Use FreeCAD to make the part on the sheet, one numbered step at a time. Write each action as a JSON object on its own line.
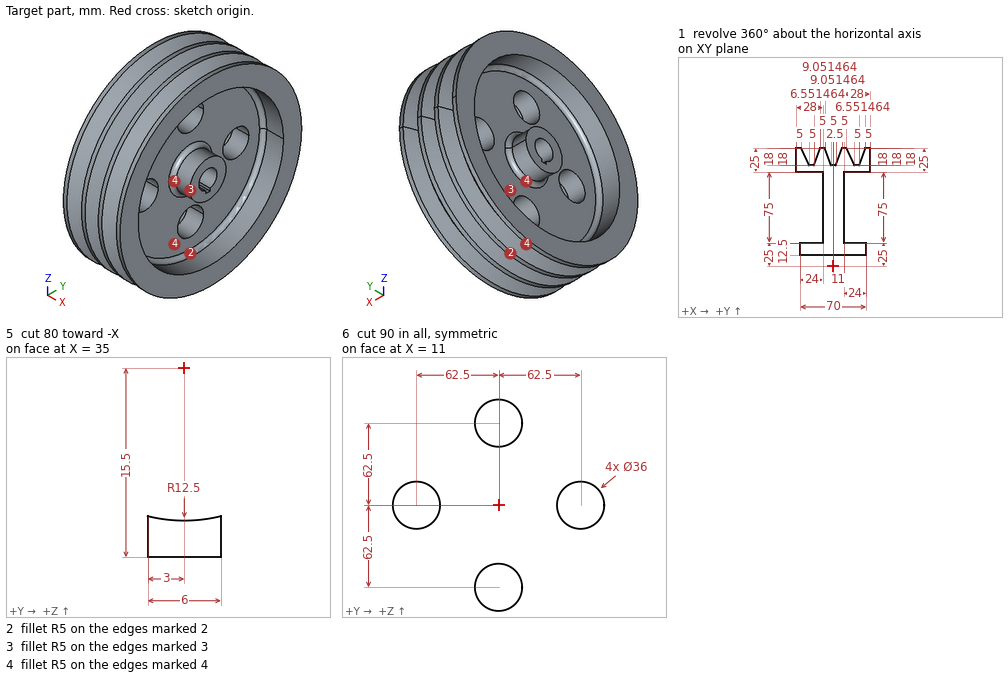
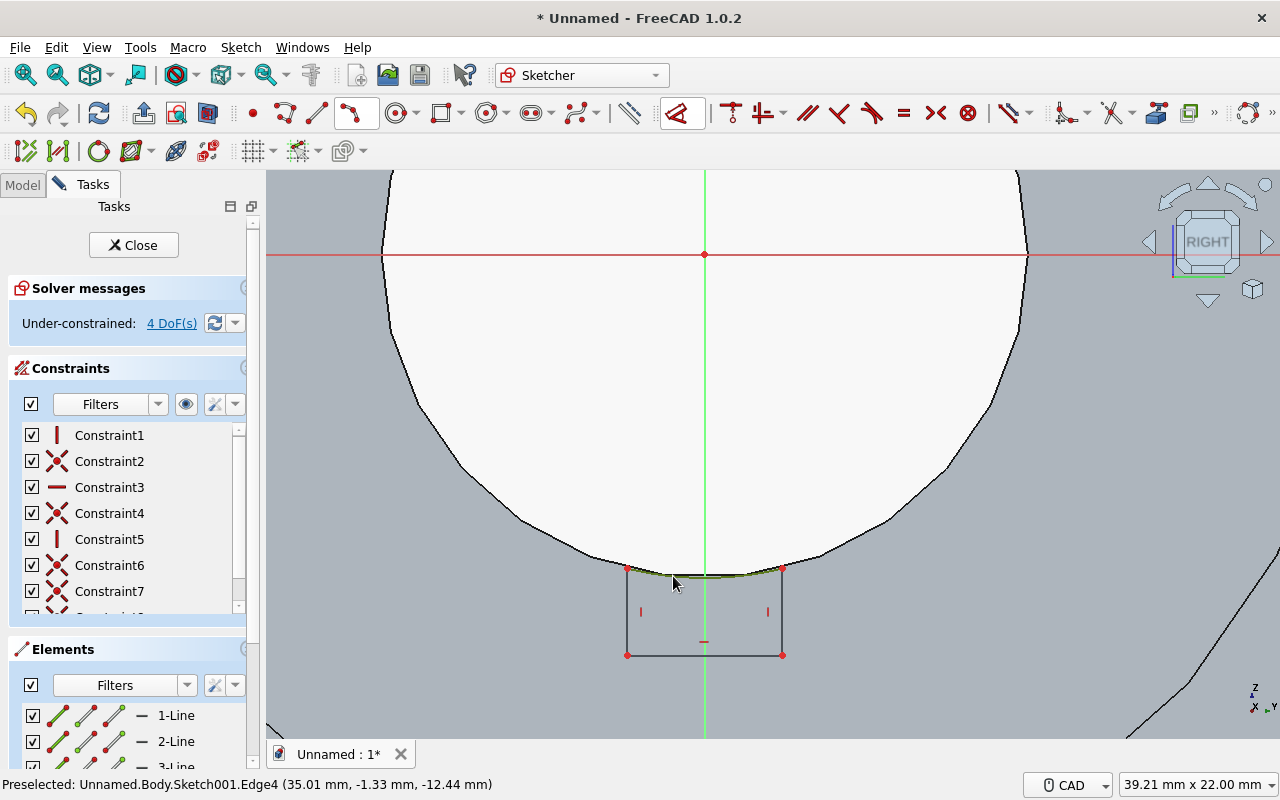
{"action": "left_click", "coordinate": [700, 114]}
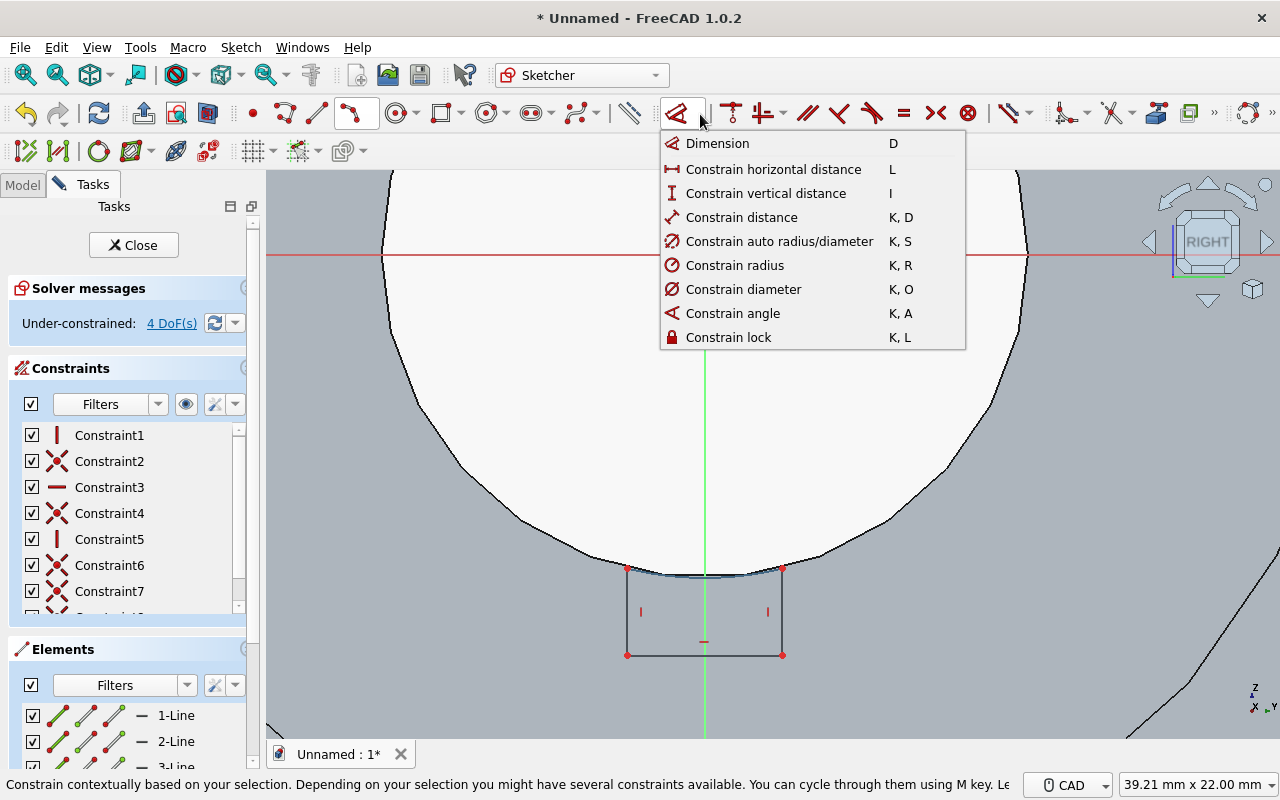
{"action": "left_click", "coordinate": [813, 265]}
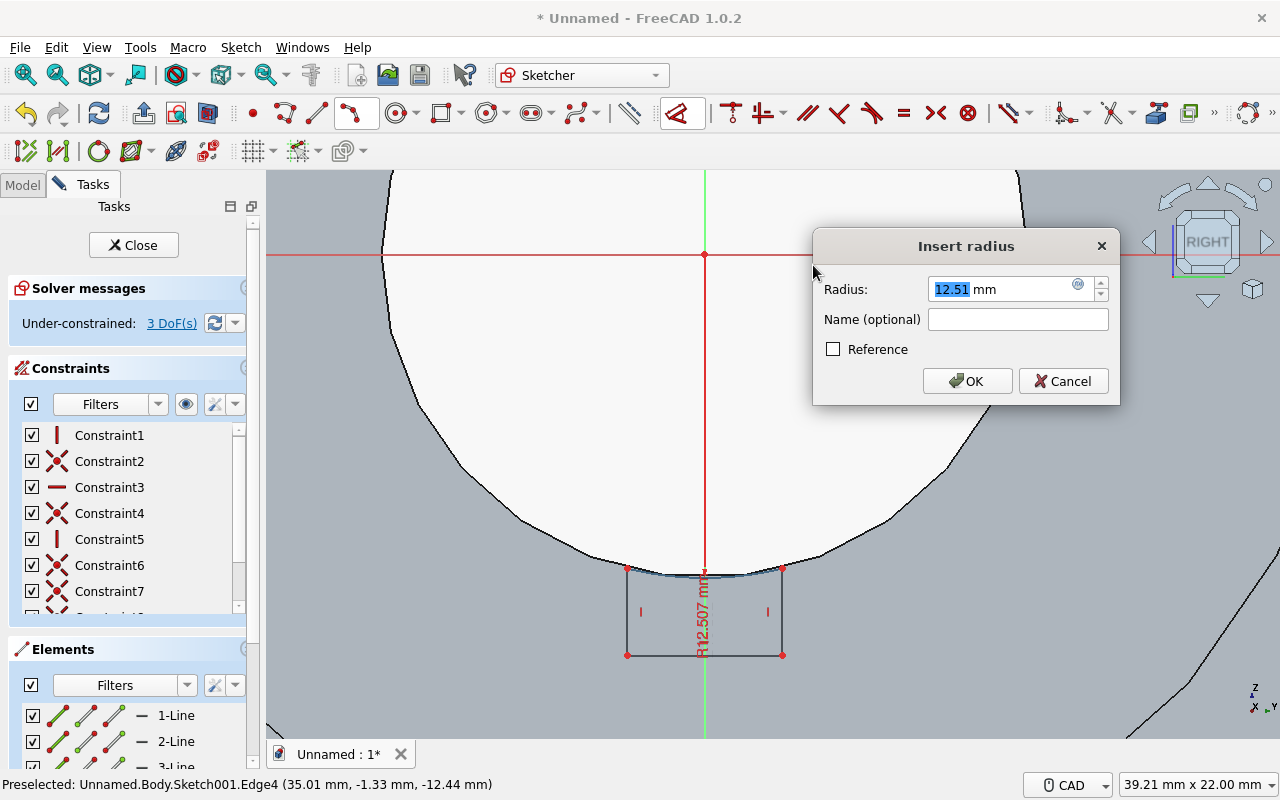
{"action": "type", "text": "12.5"}
{"action": "key", "text": "Return"}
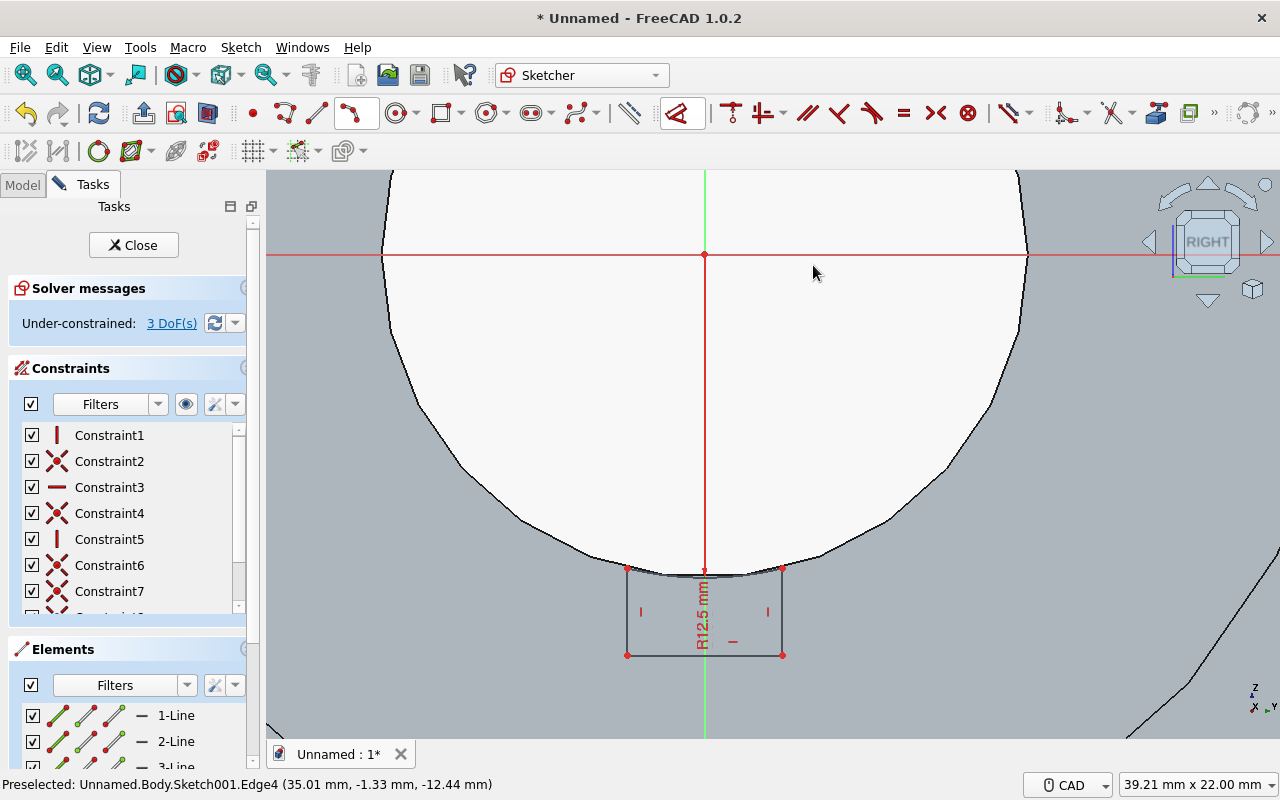
{"action": "left_click", "coordinate": [674, 656]}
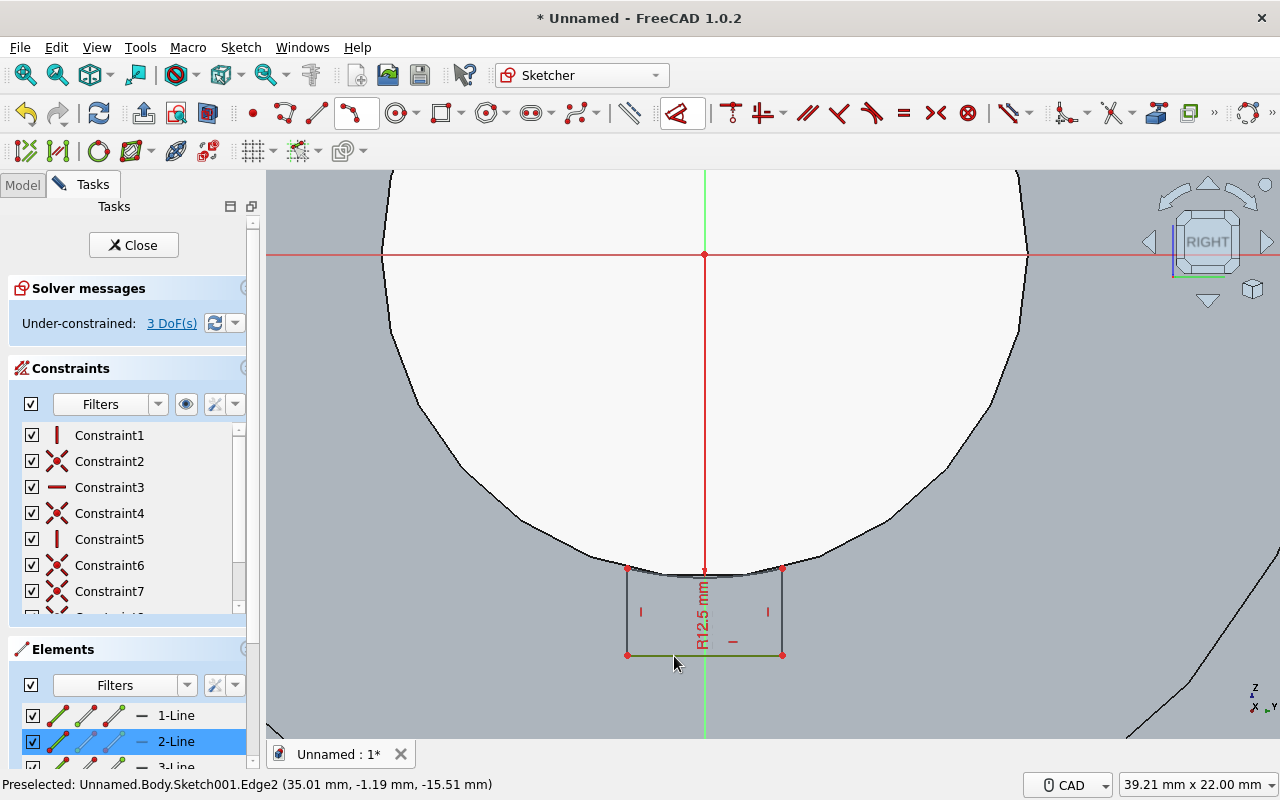
{"action": "left_click", "coordinate": [700, 114]}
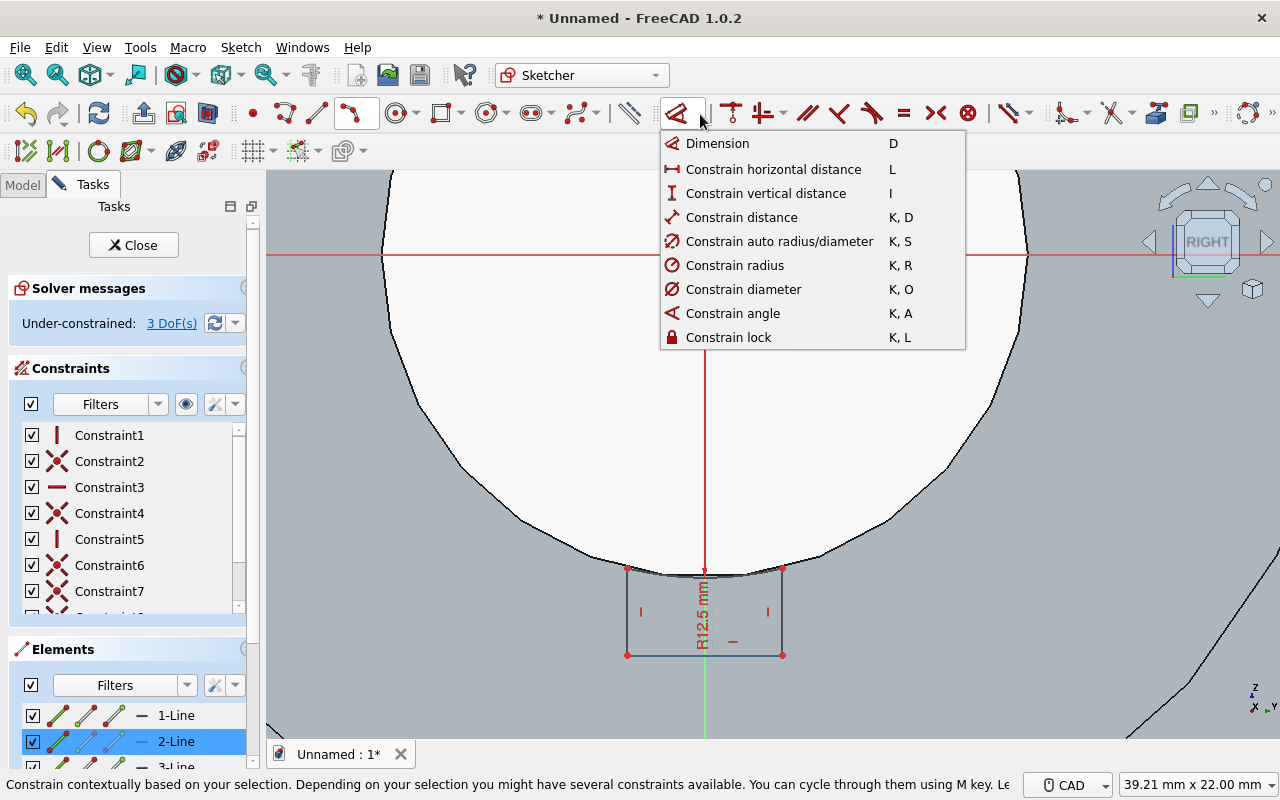
{"action": "left_click", "coordinate": [813, 169]}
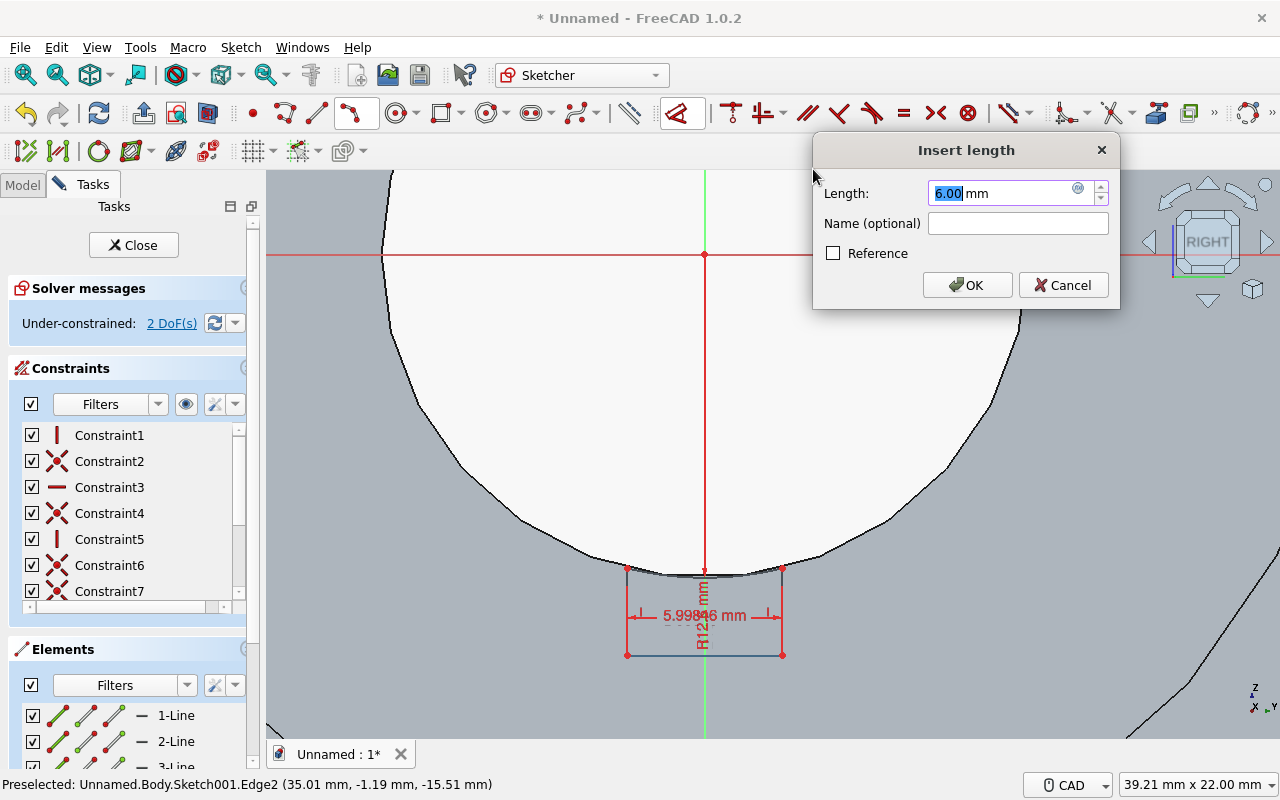
{"action": "type", "text": "6"}
{"action": "key", "text": "Return"}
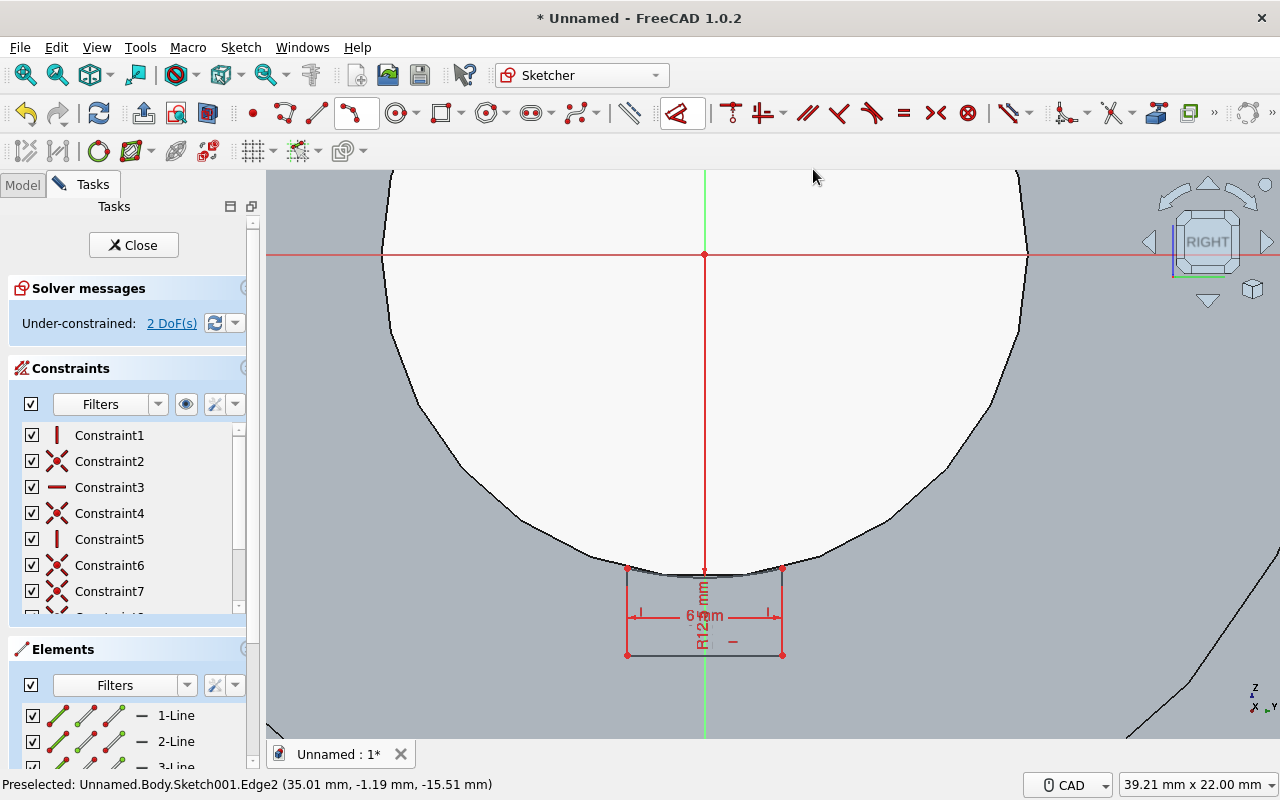
{"action": "left_click", "coordinate": [627, 568]}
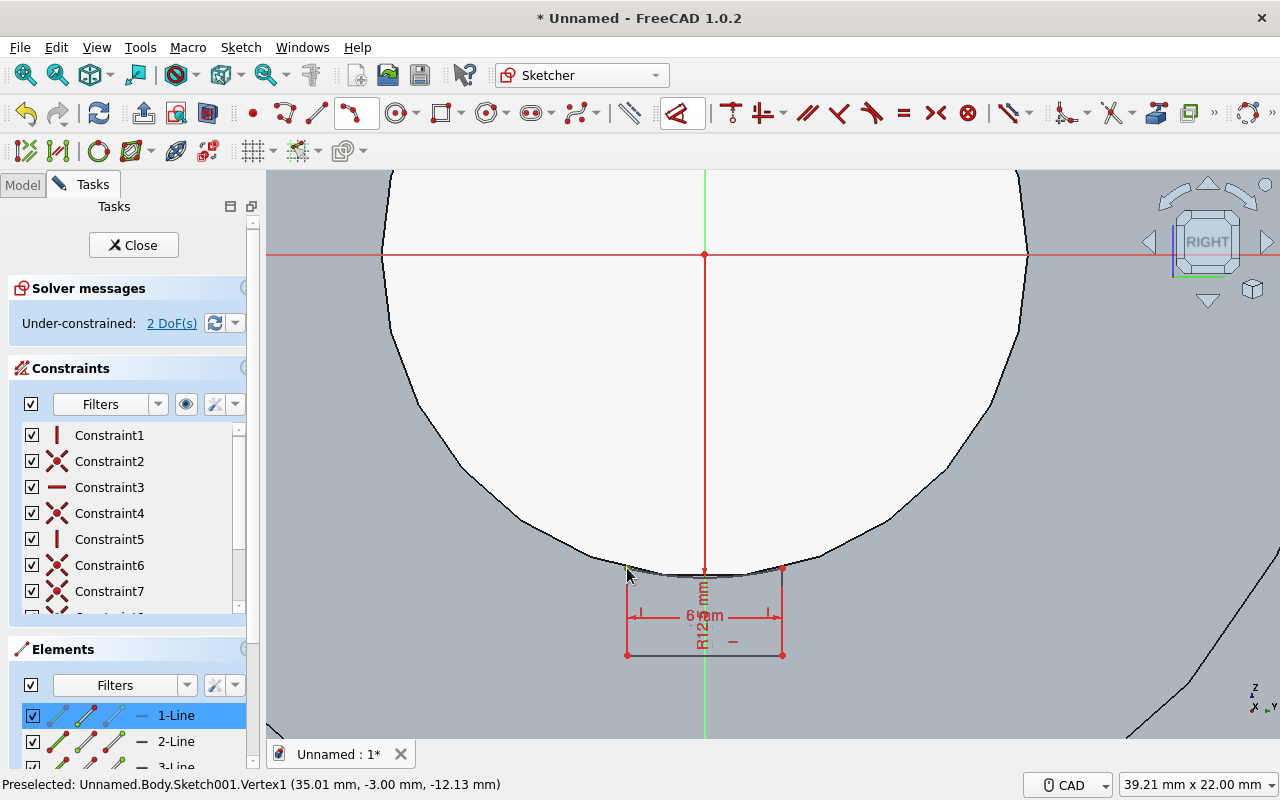
{"action": "key", "text": "l"}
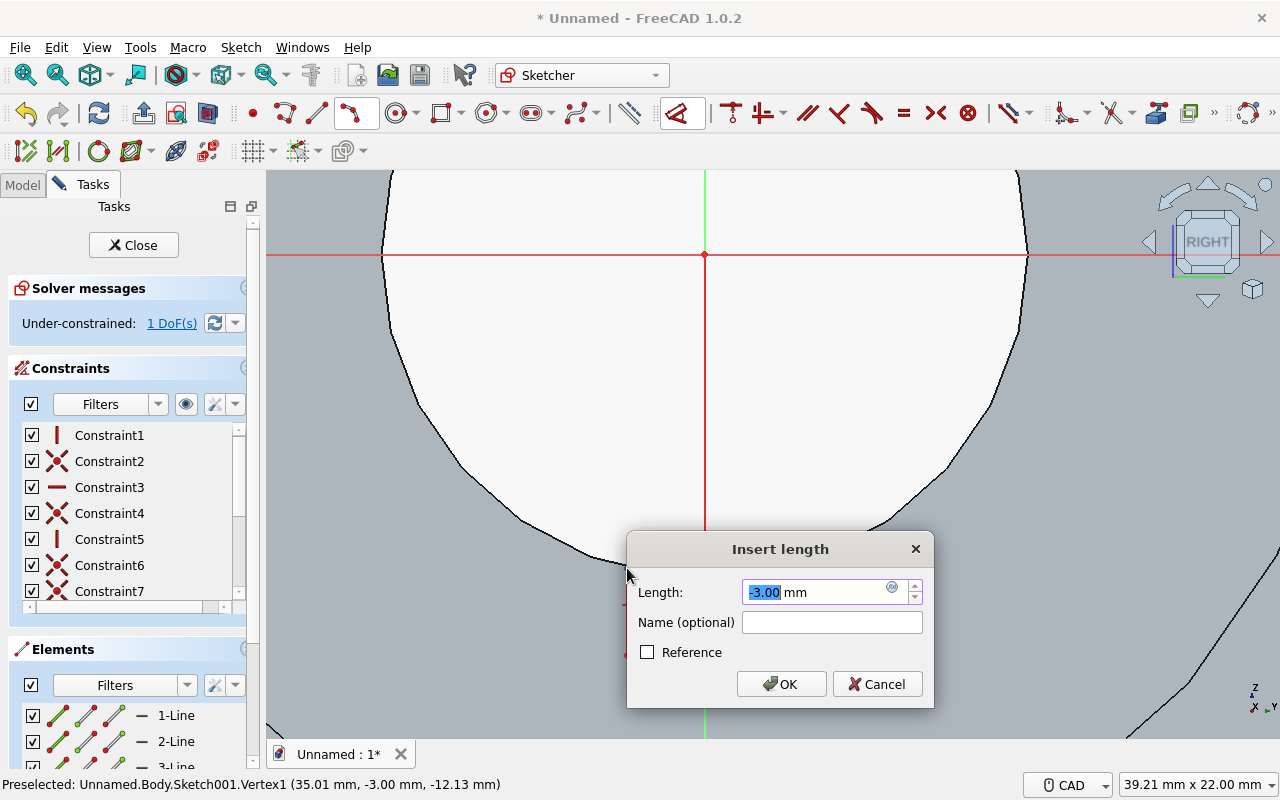
{"action": "type", "text": "-3"}
{"action": "key", "text": "Return"}